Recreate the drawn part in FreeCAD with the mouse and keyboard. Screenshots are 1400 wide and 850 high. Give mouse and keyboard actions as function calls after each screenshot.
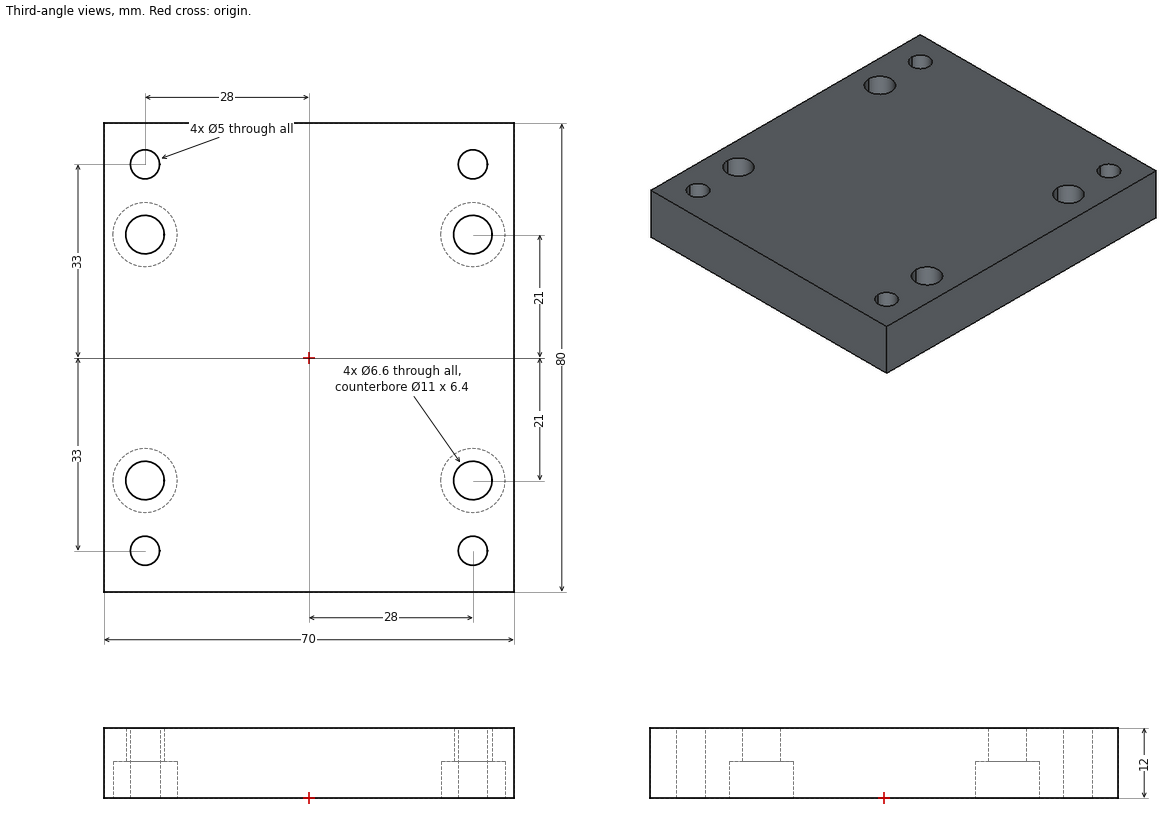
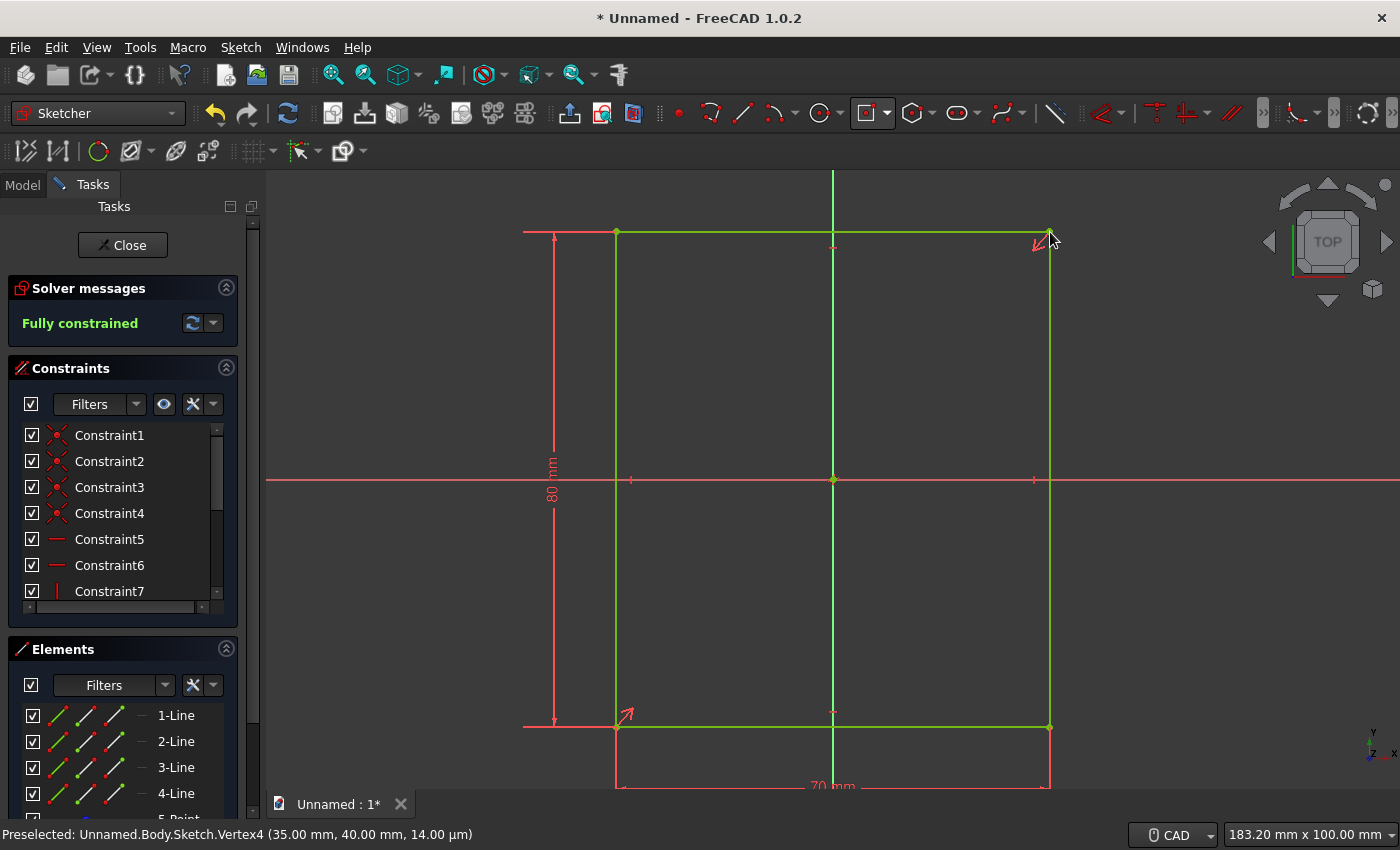
click(123, 245)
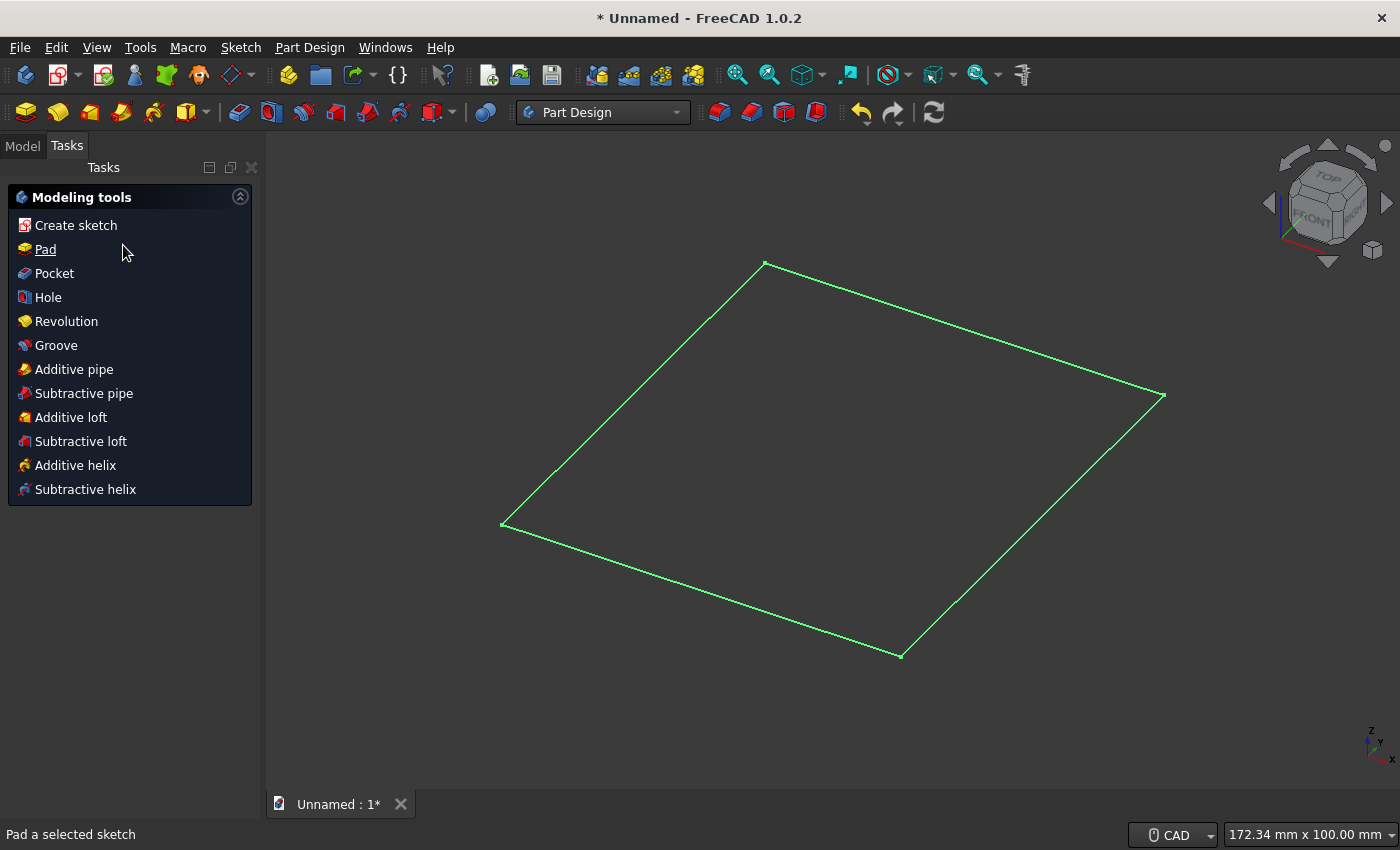
click(26, 112)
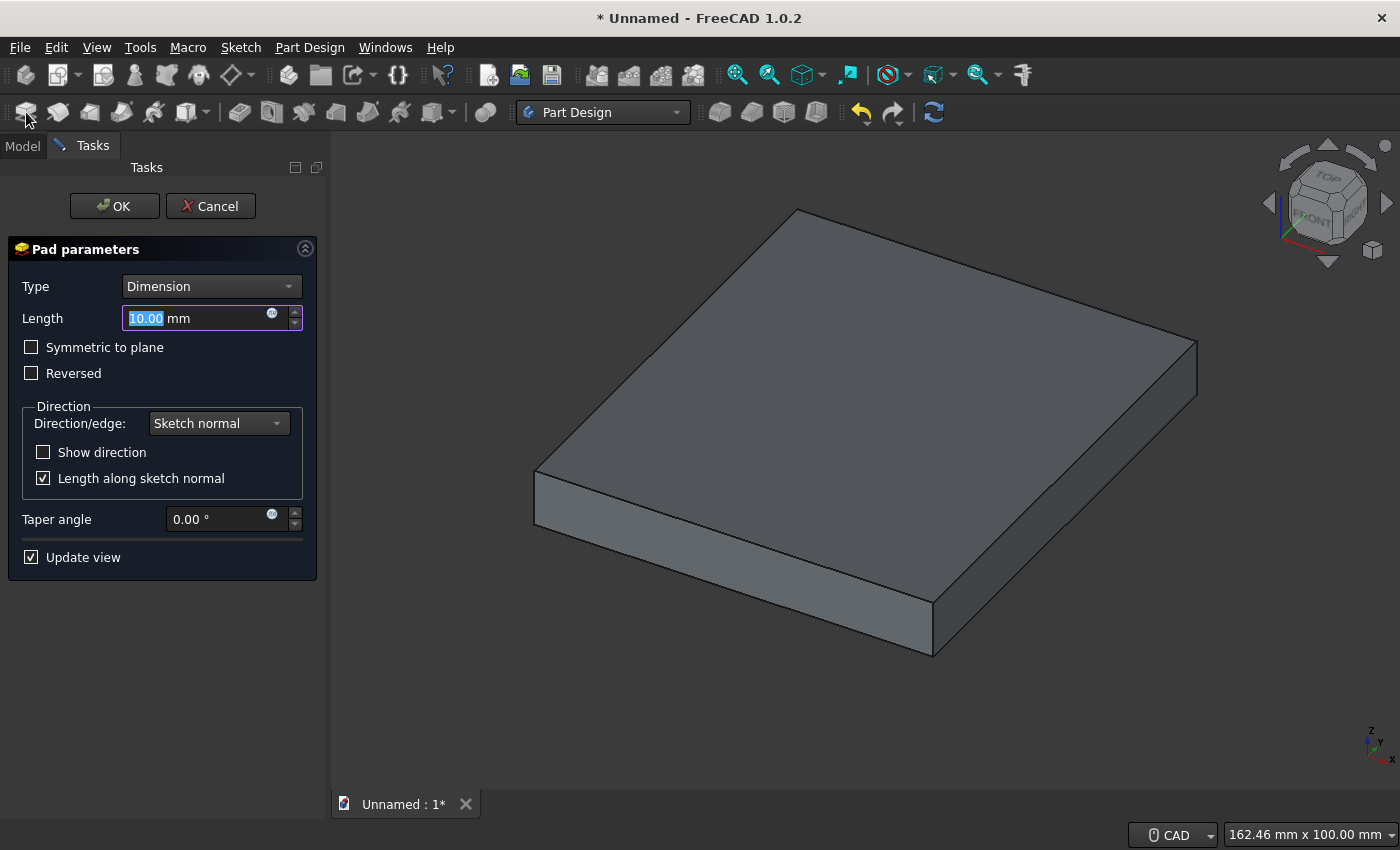
text(12)
key(Tab)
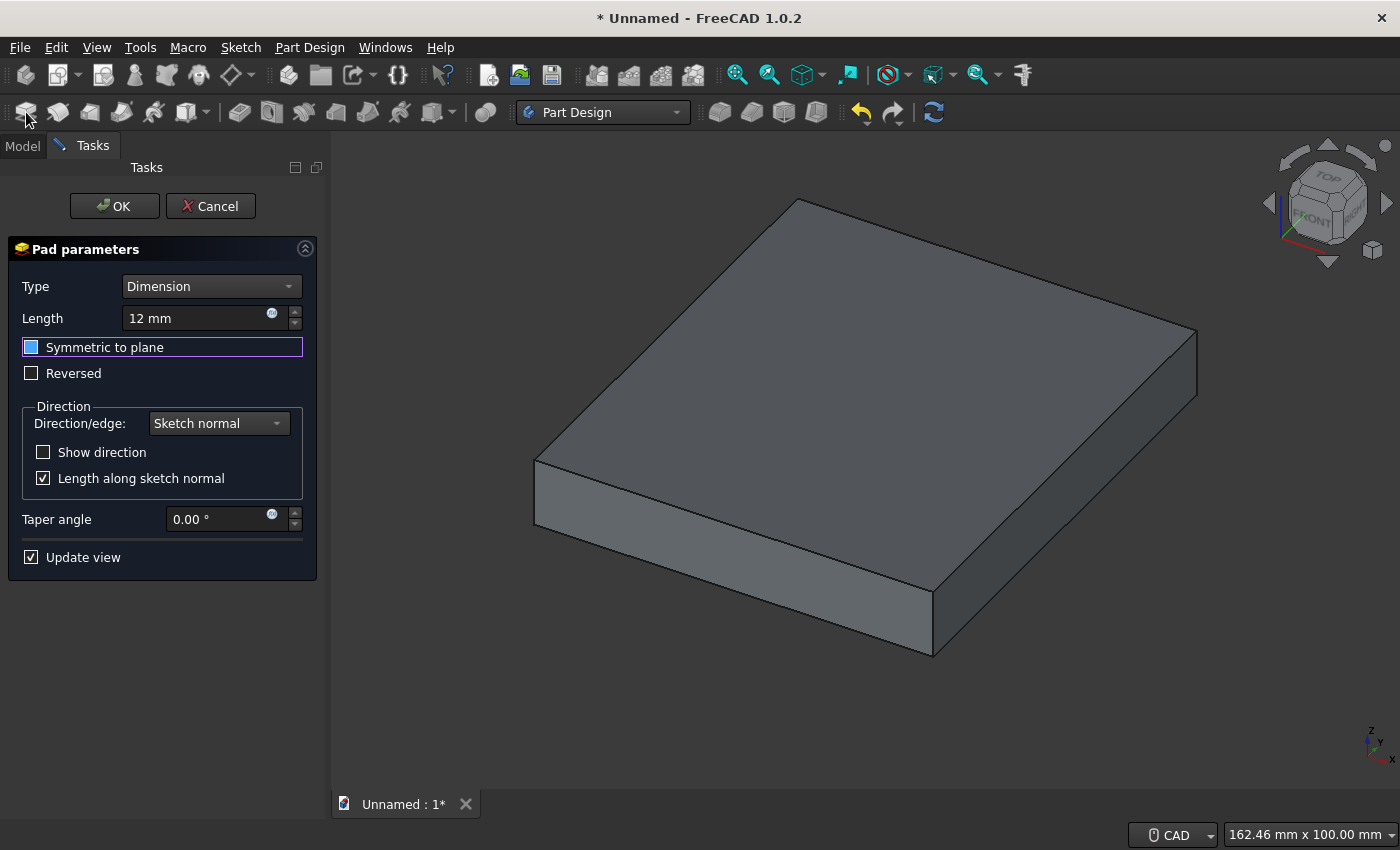
click(115, 206)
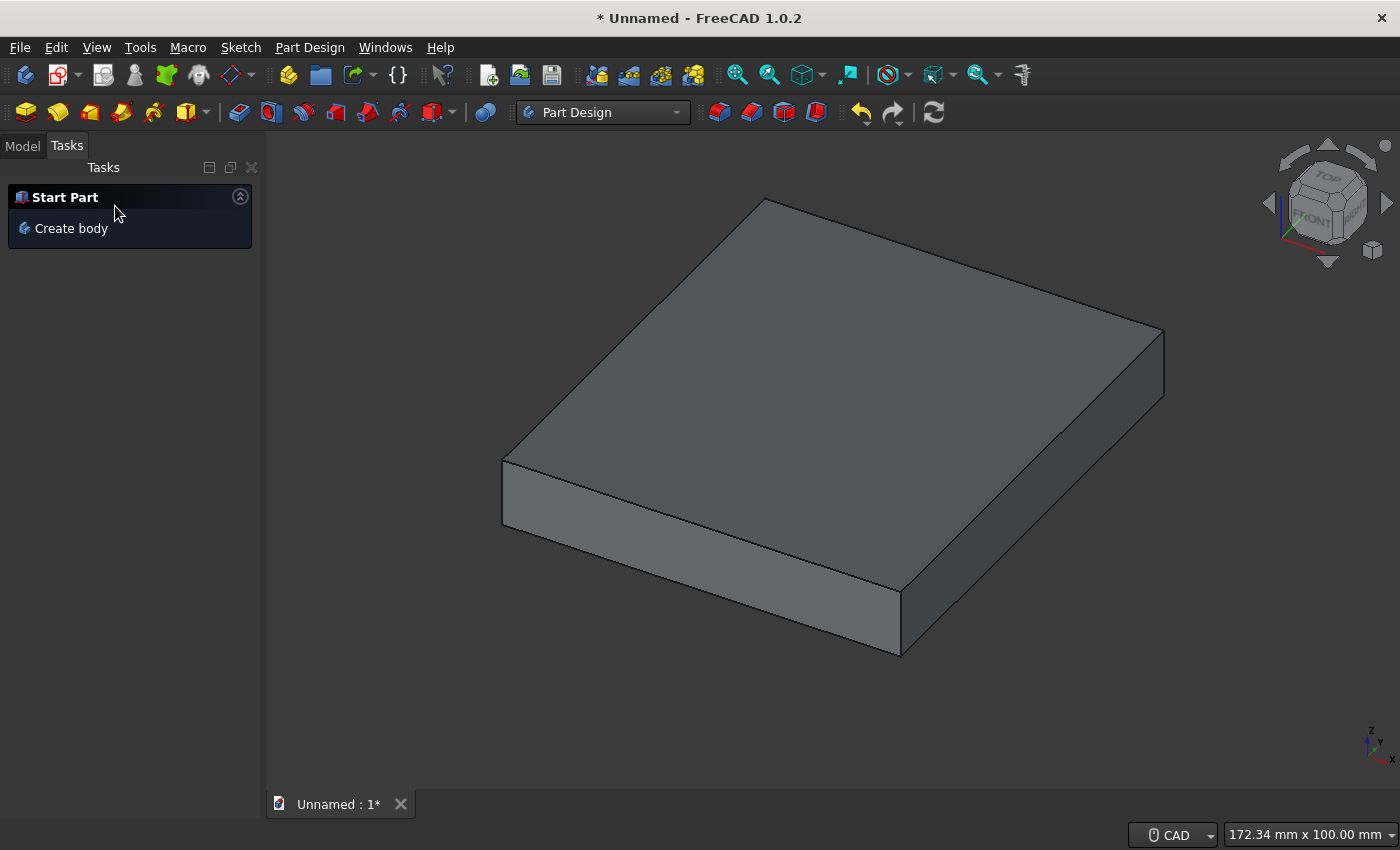
key(5)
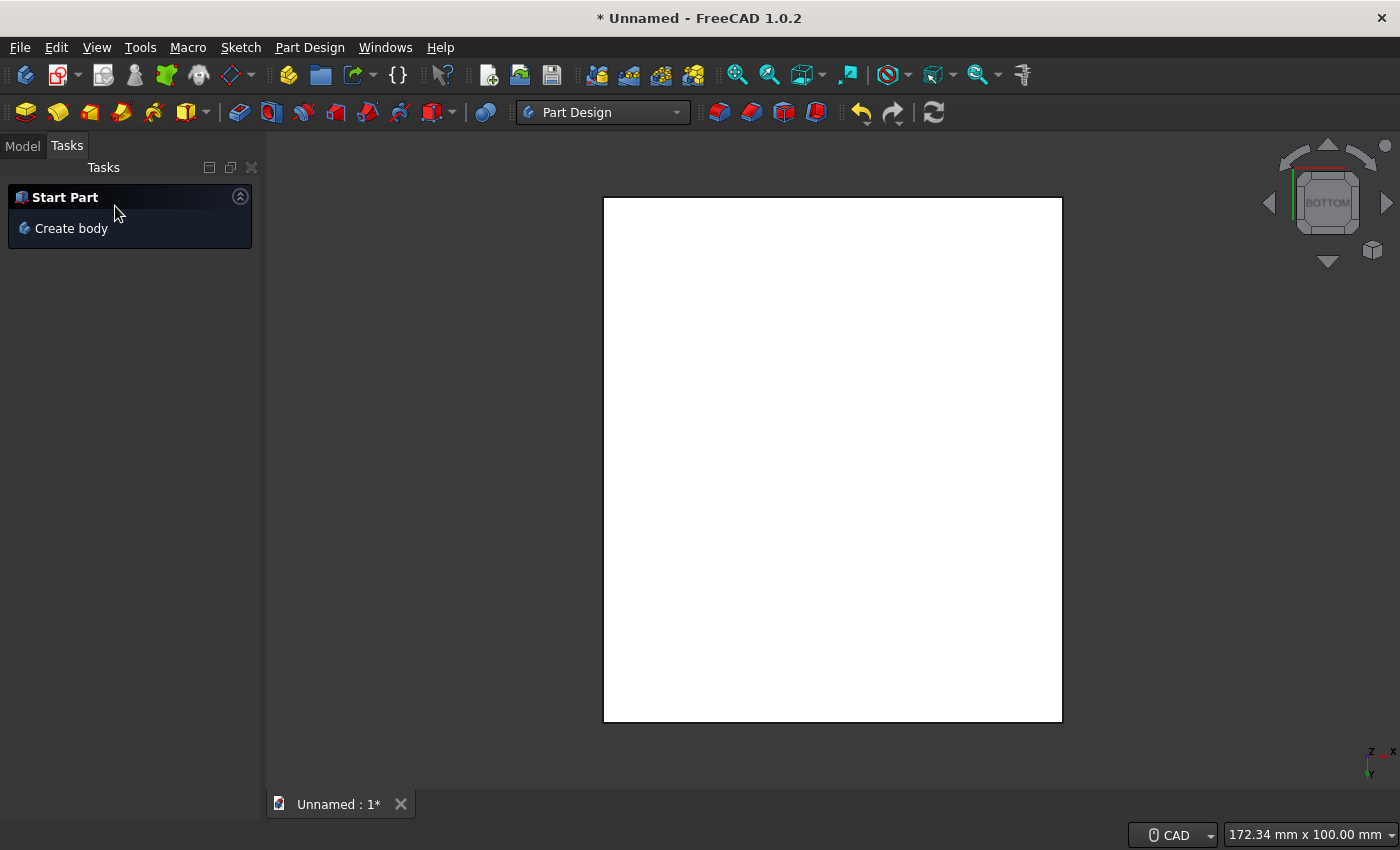
click(833, 459)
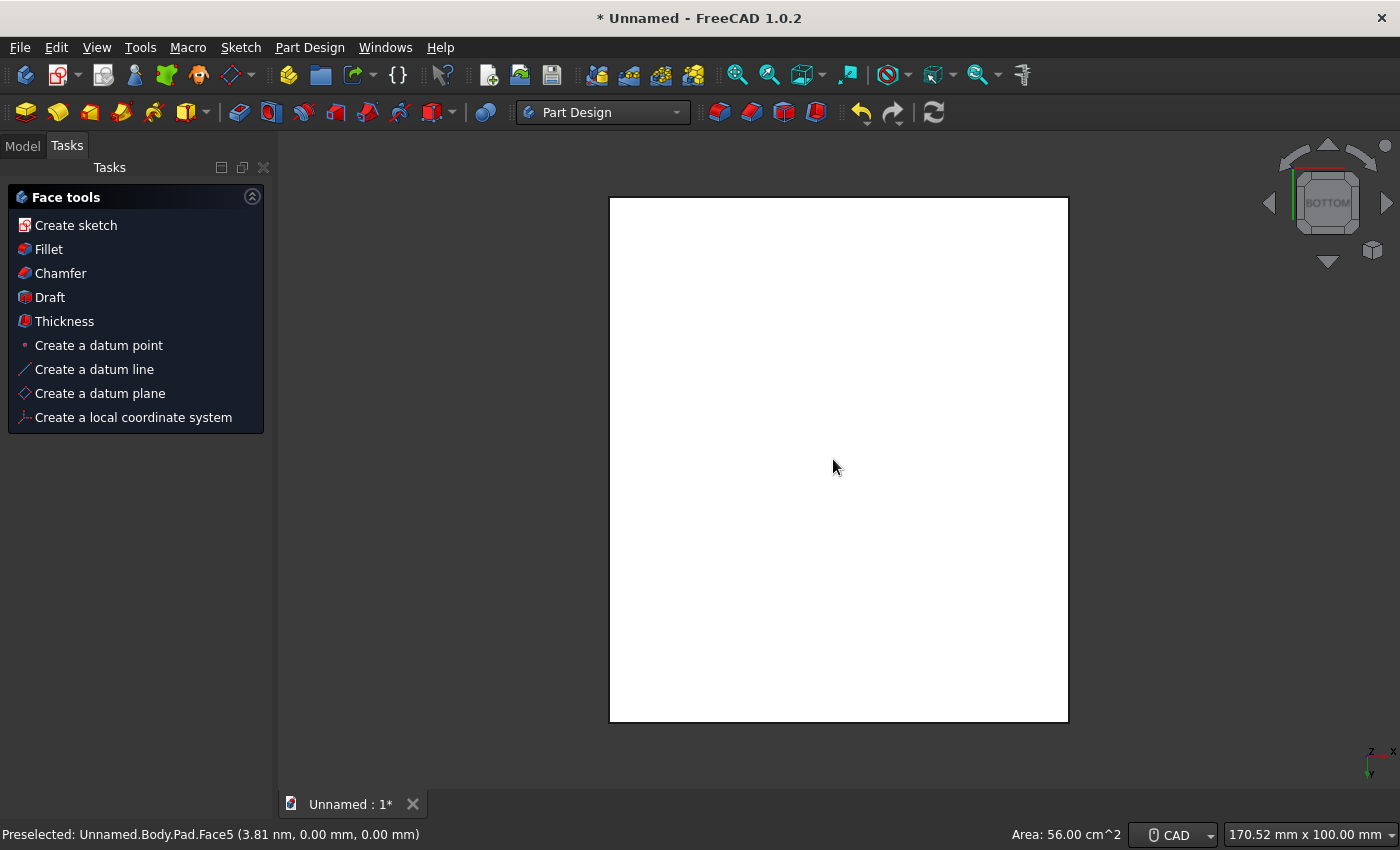
click(58, 76)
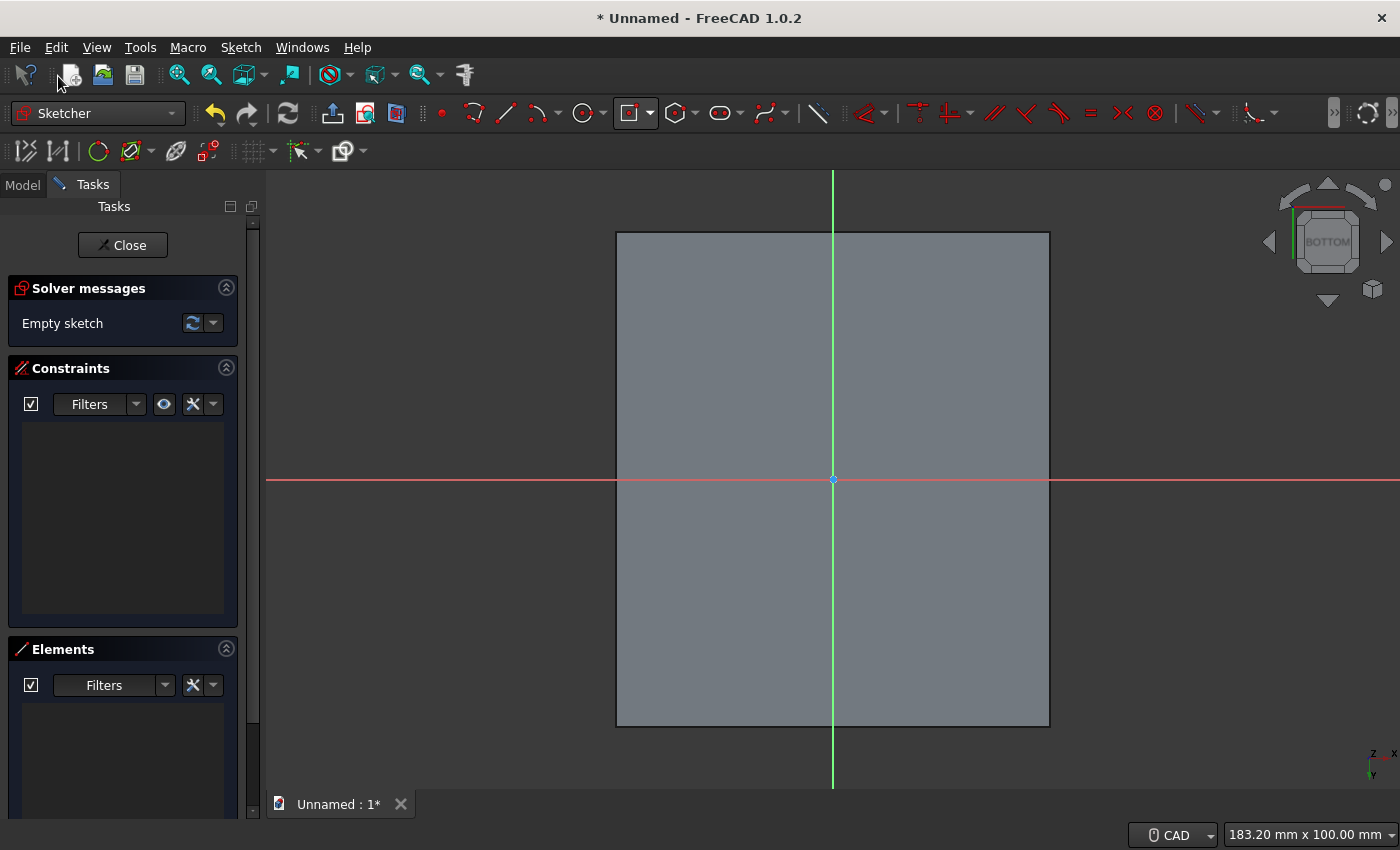
click(584, 114)